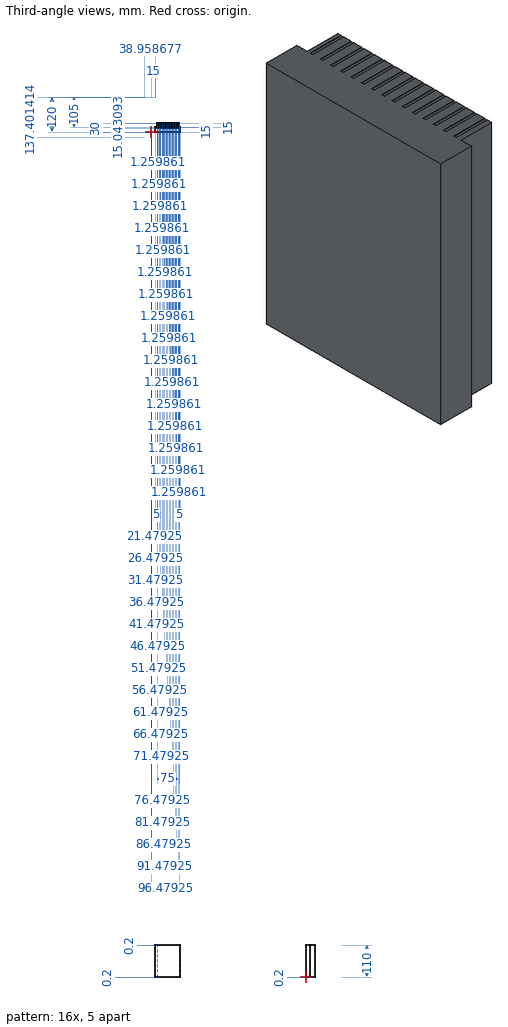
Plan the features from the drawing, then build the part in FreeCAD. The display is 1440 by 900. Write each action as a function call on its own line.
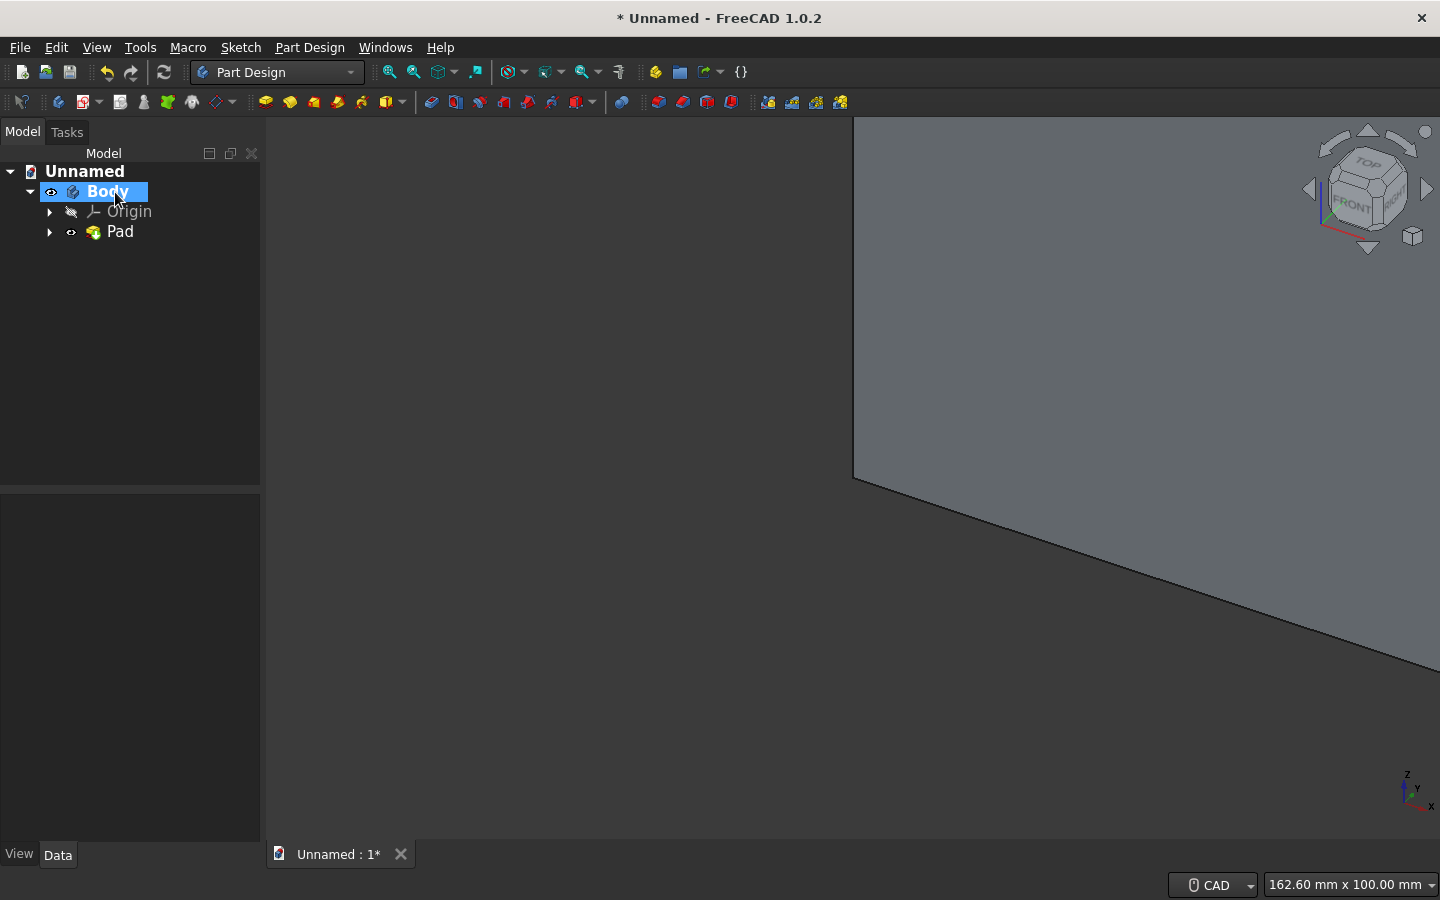
key(v)
key(f)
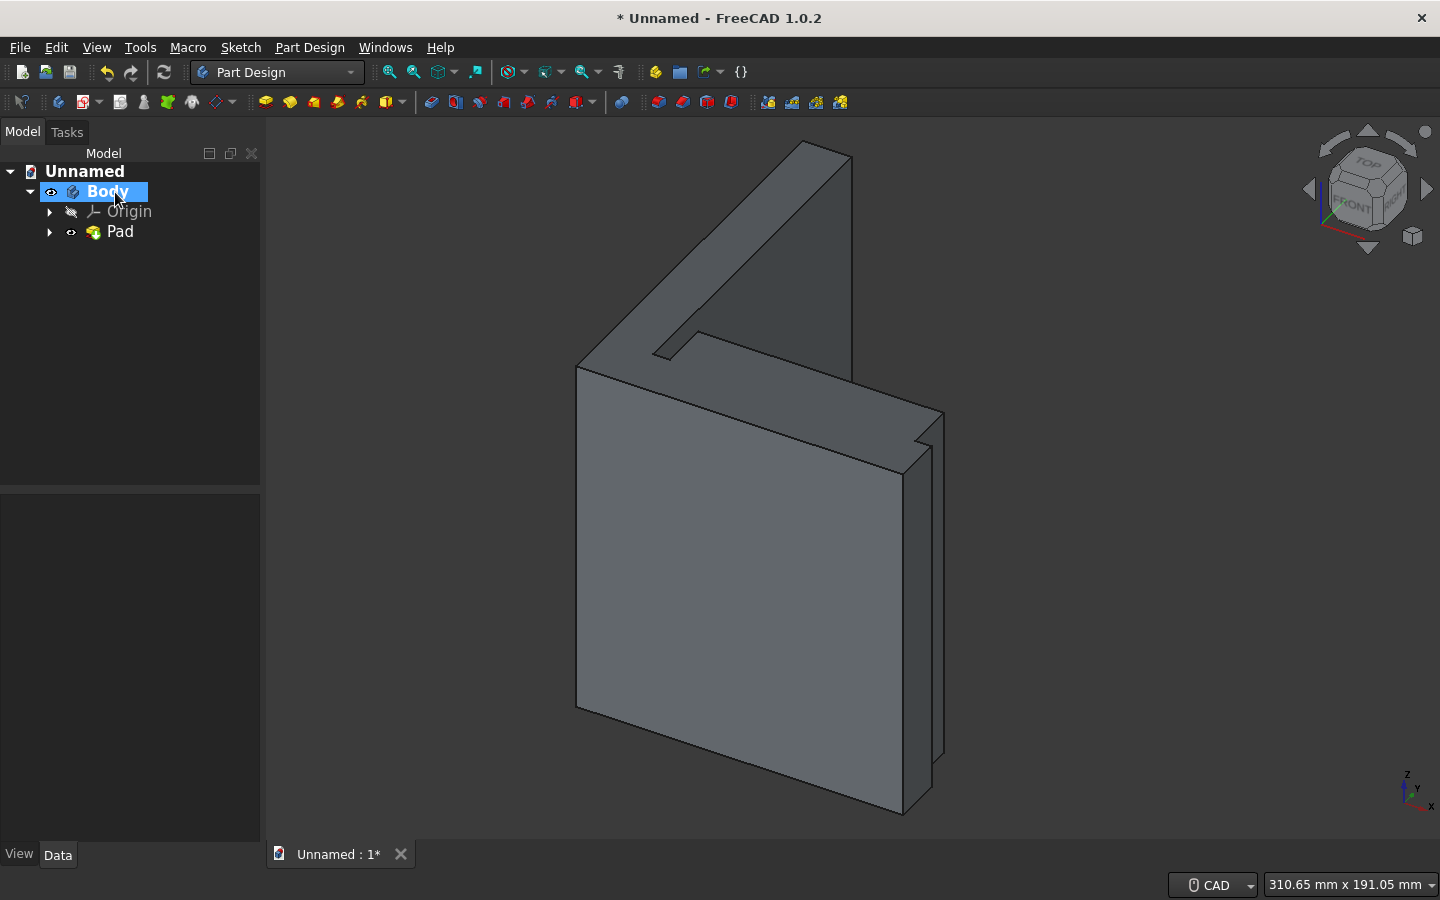
click(849, 434)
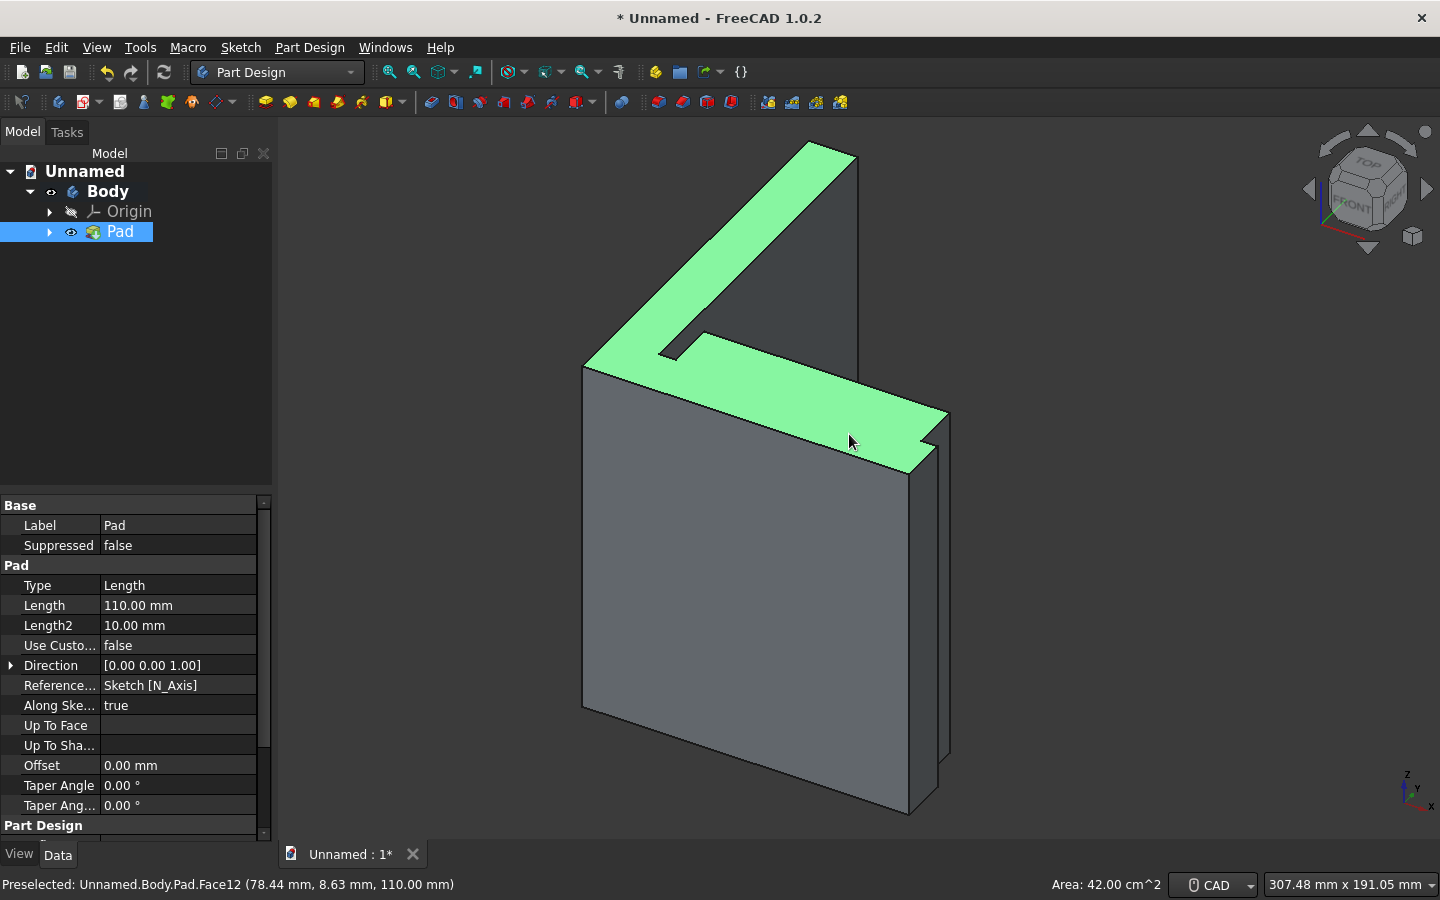
click(84, 102)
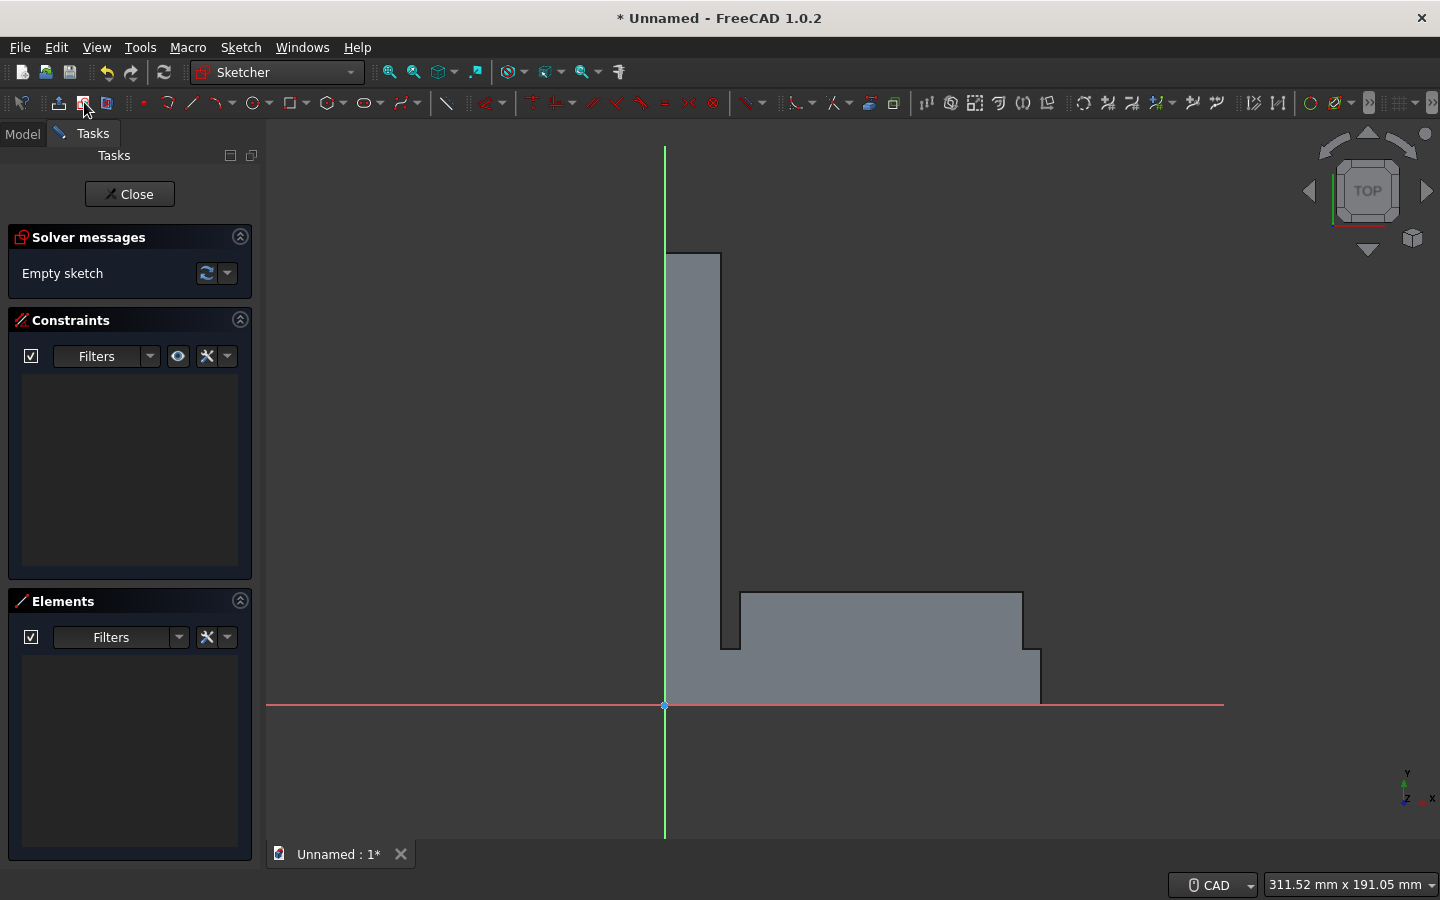
scroll(682, 704, up, 7)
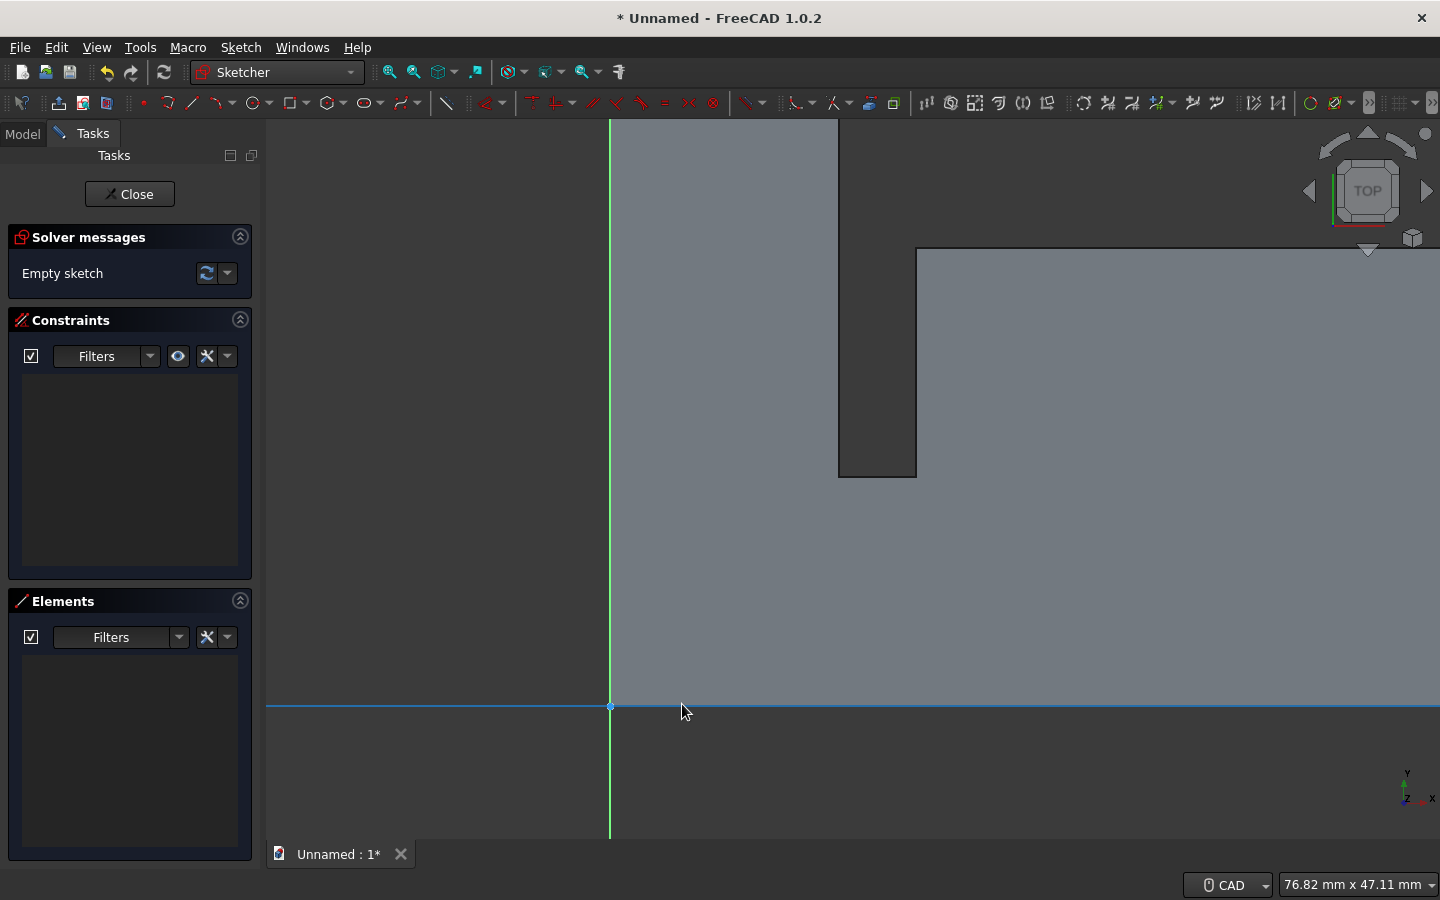
click(290, 104)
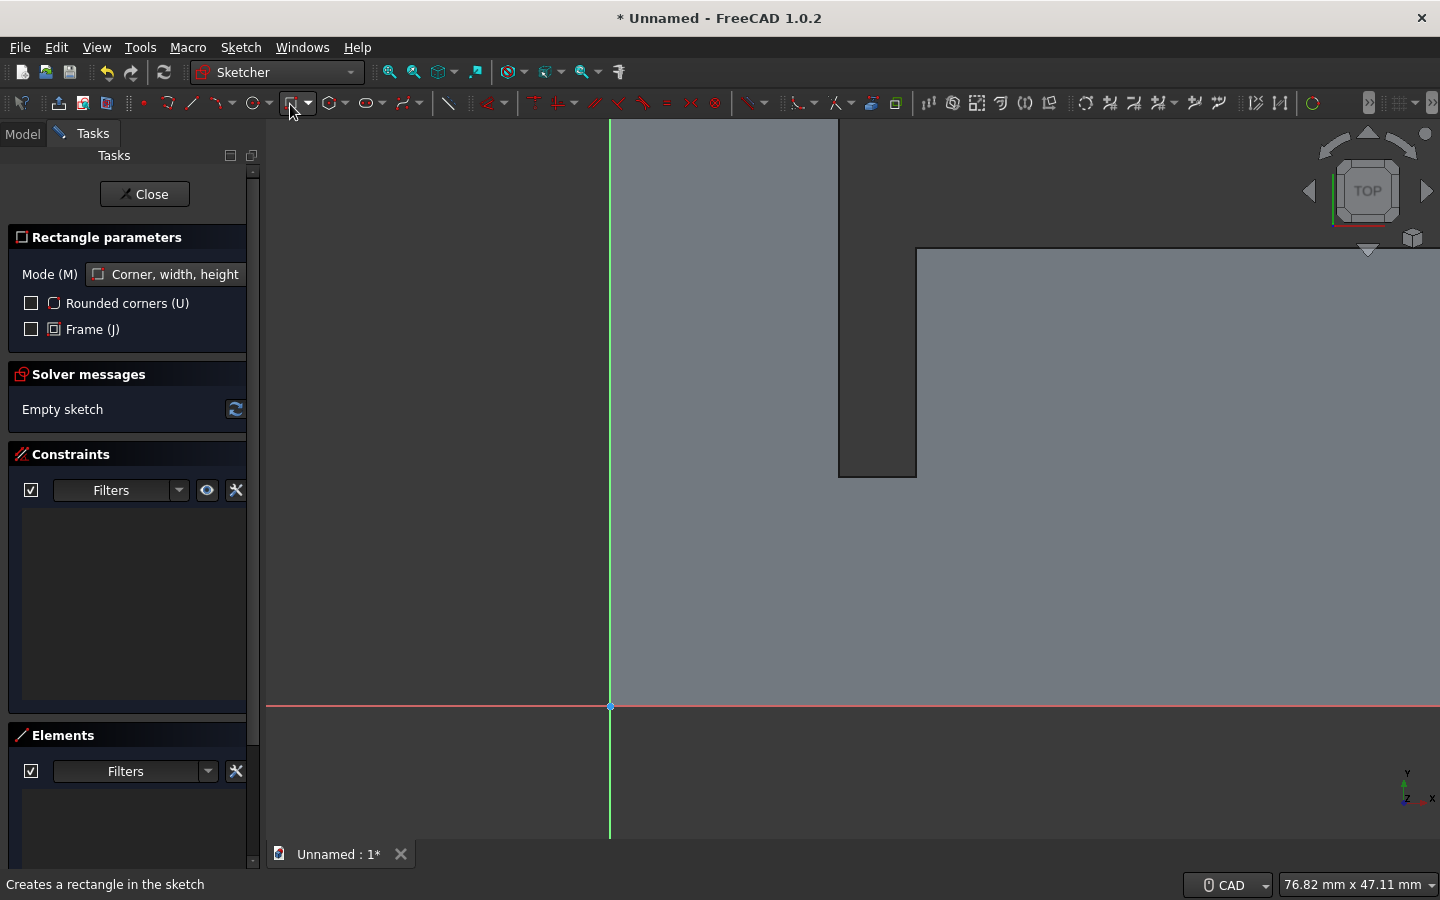
click(938, 248)
click(958, 477)
key(Escape)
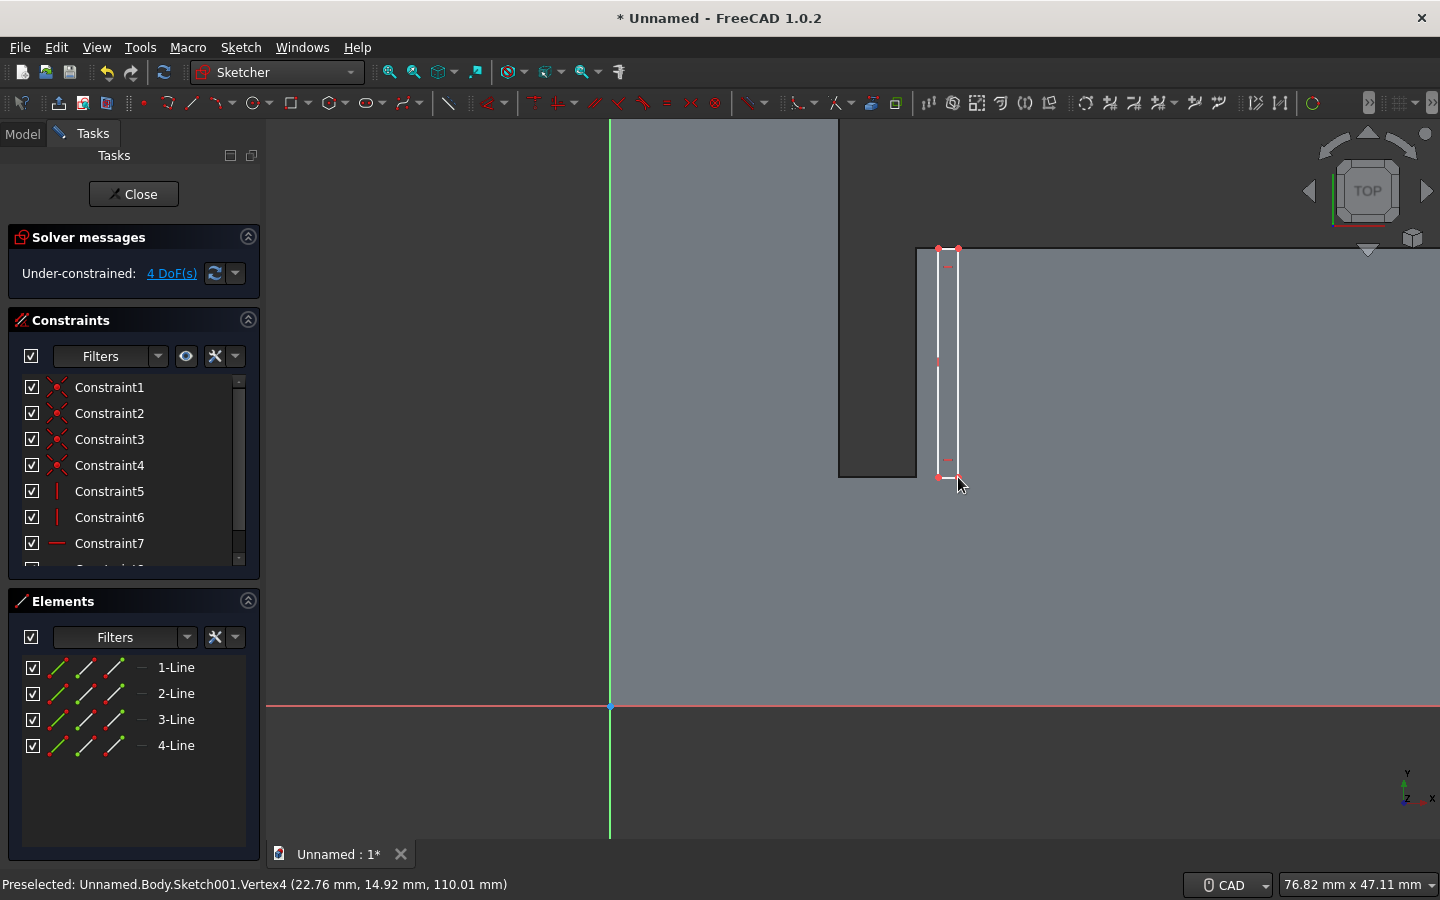
click(488, 104)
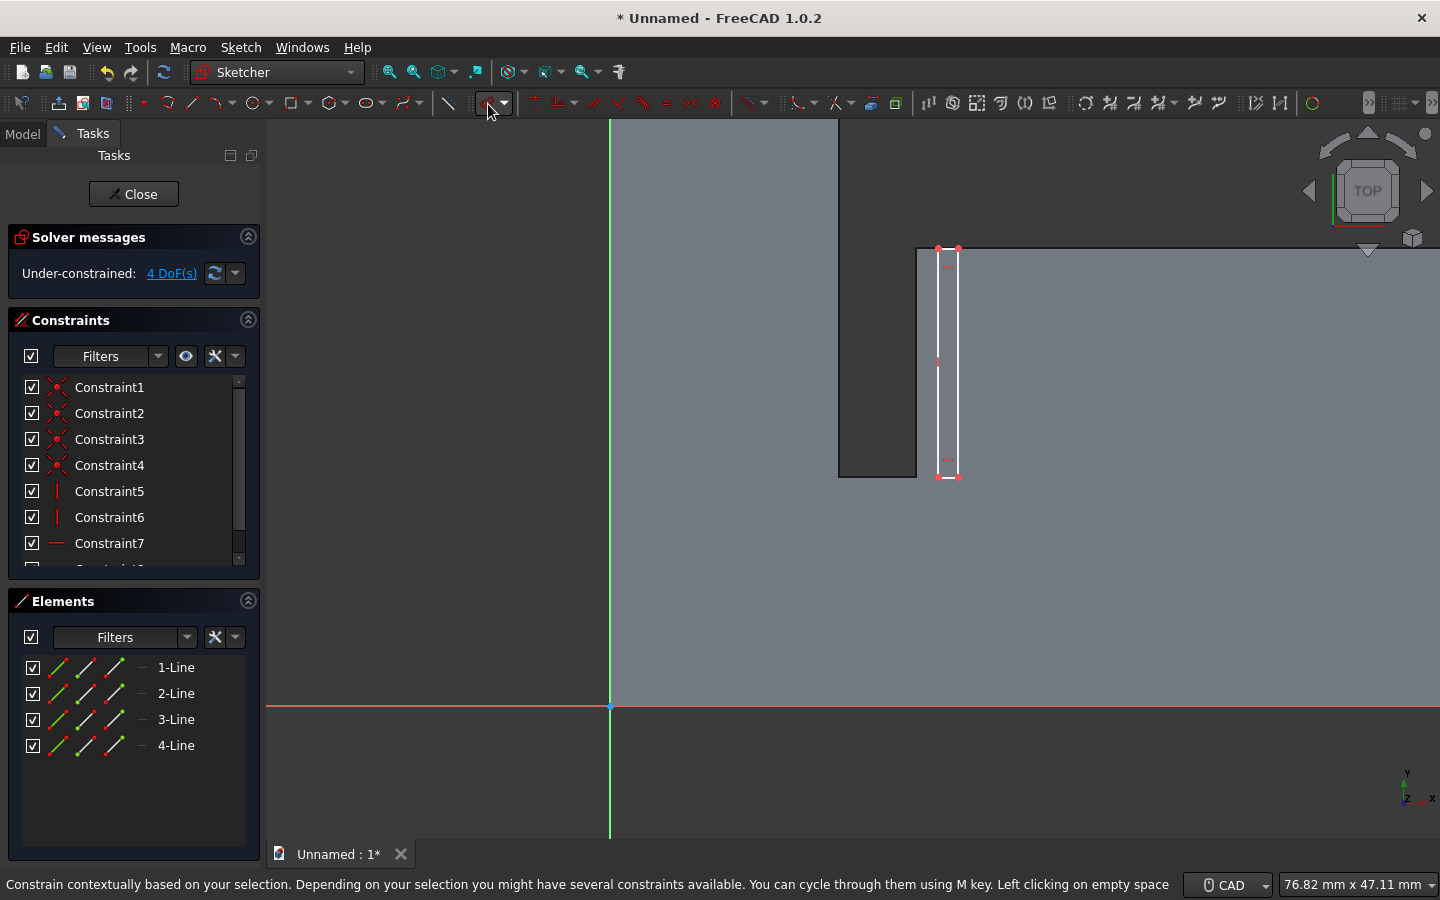
click(938, 249)
click(576, 478)